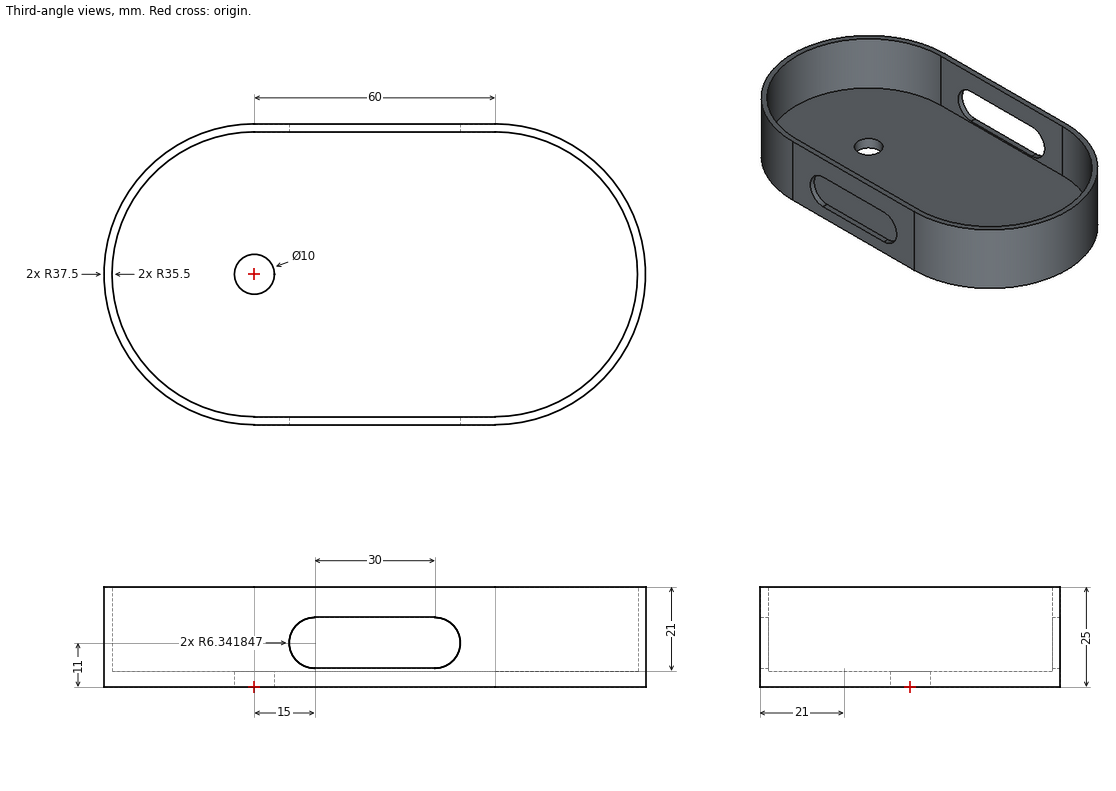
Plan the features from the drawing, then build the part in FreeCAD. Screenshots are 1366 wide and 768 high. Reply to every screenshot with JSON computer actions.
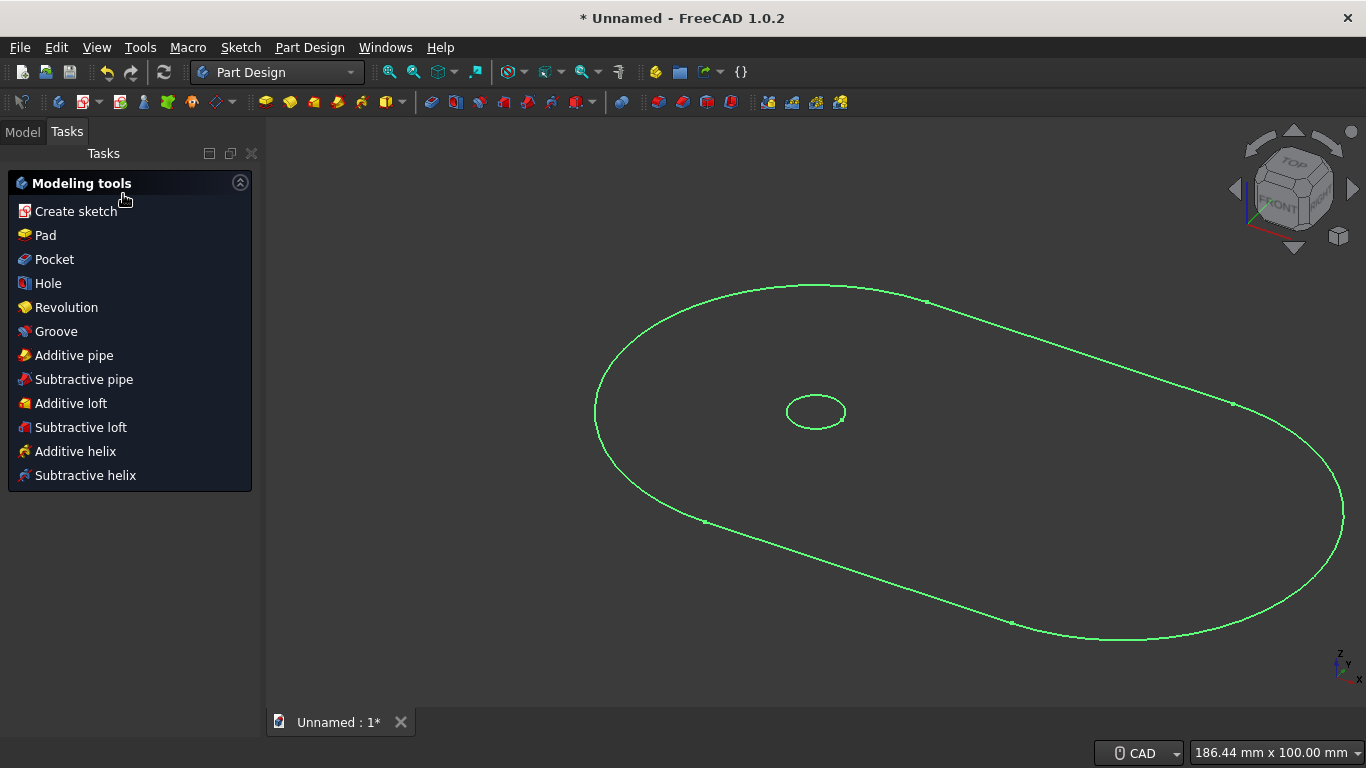
{"action": "left_click", "coordinate": [266, 102]}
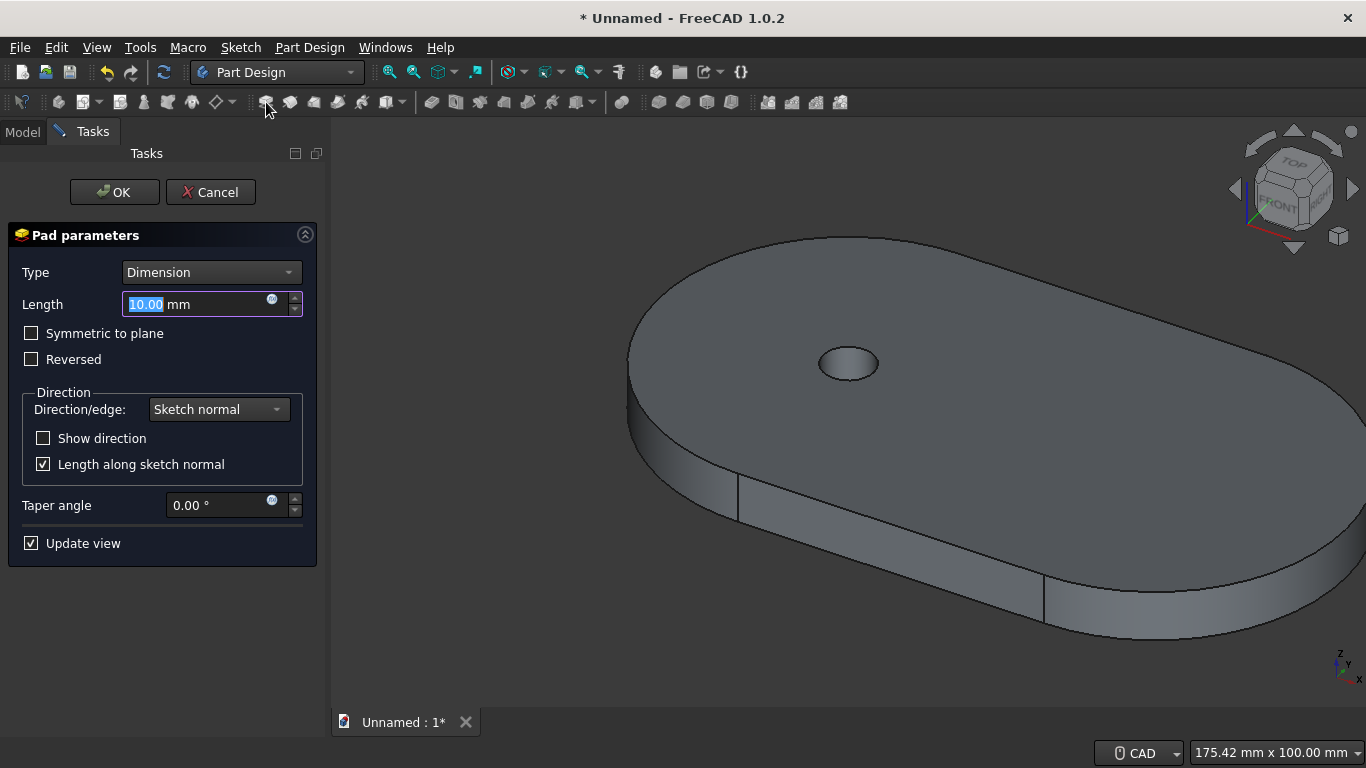
{"action": "type", "text": "25"}
{"action": "key", "text": "Tab"}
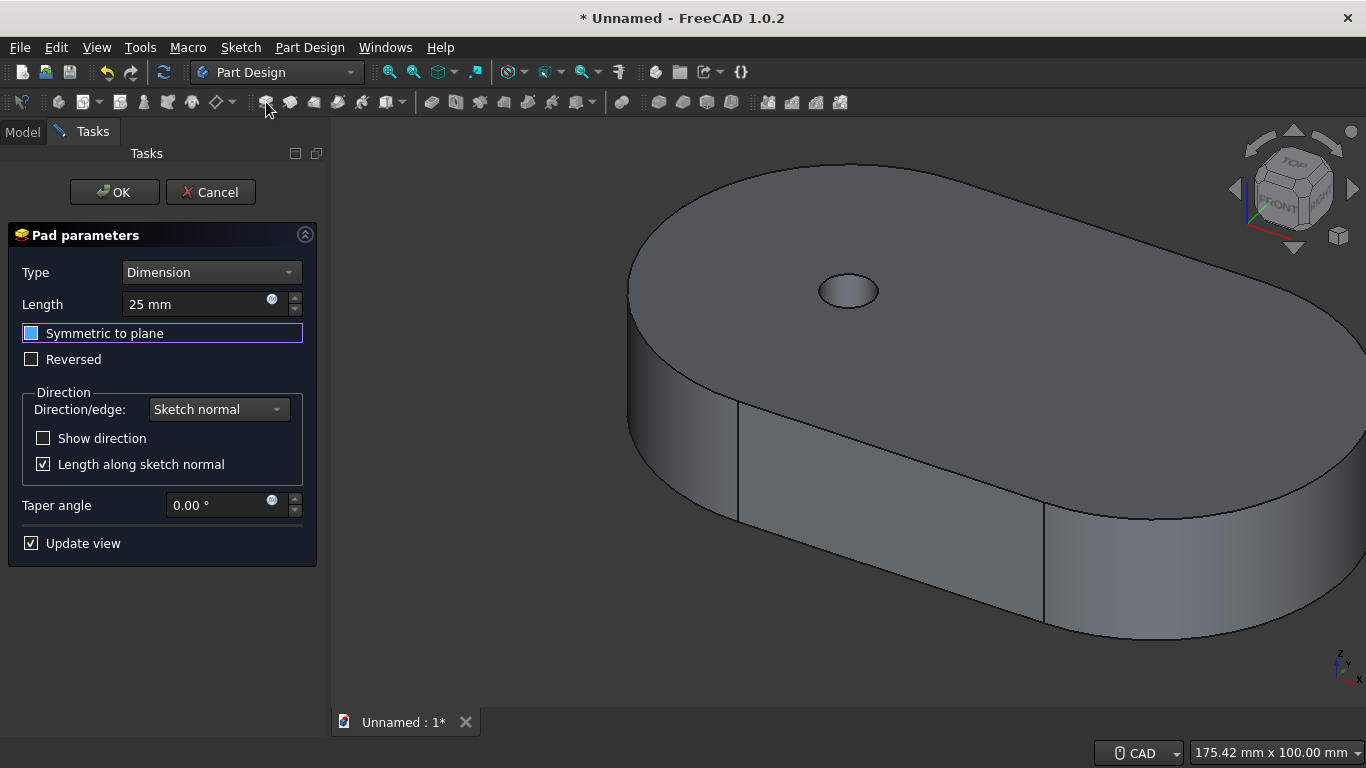
{"action": "left_click", "coordinate": [115, 192]}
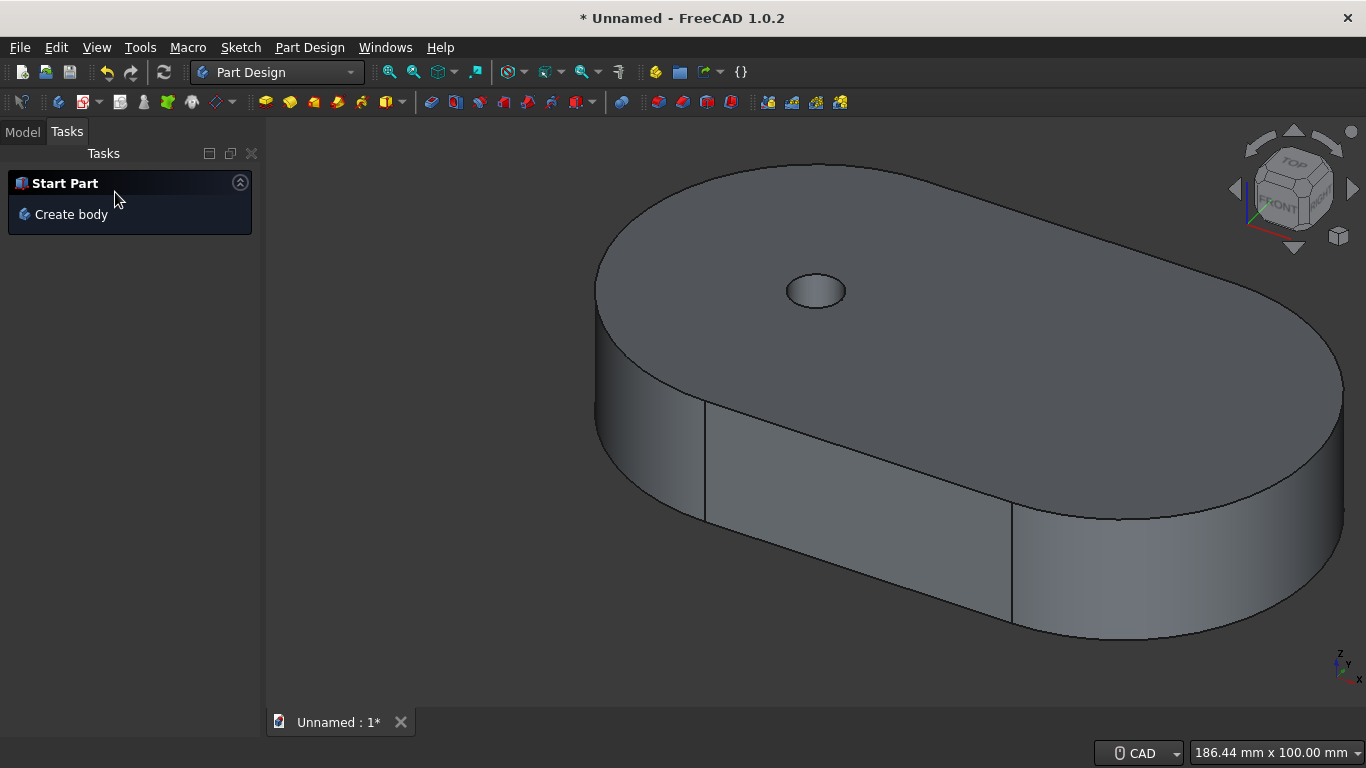
{"action": "left_click", "coordinate": [390, 72]}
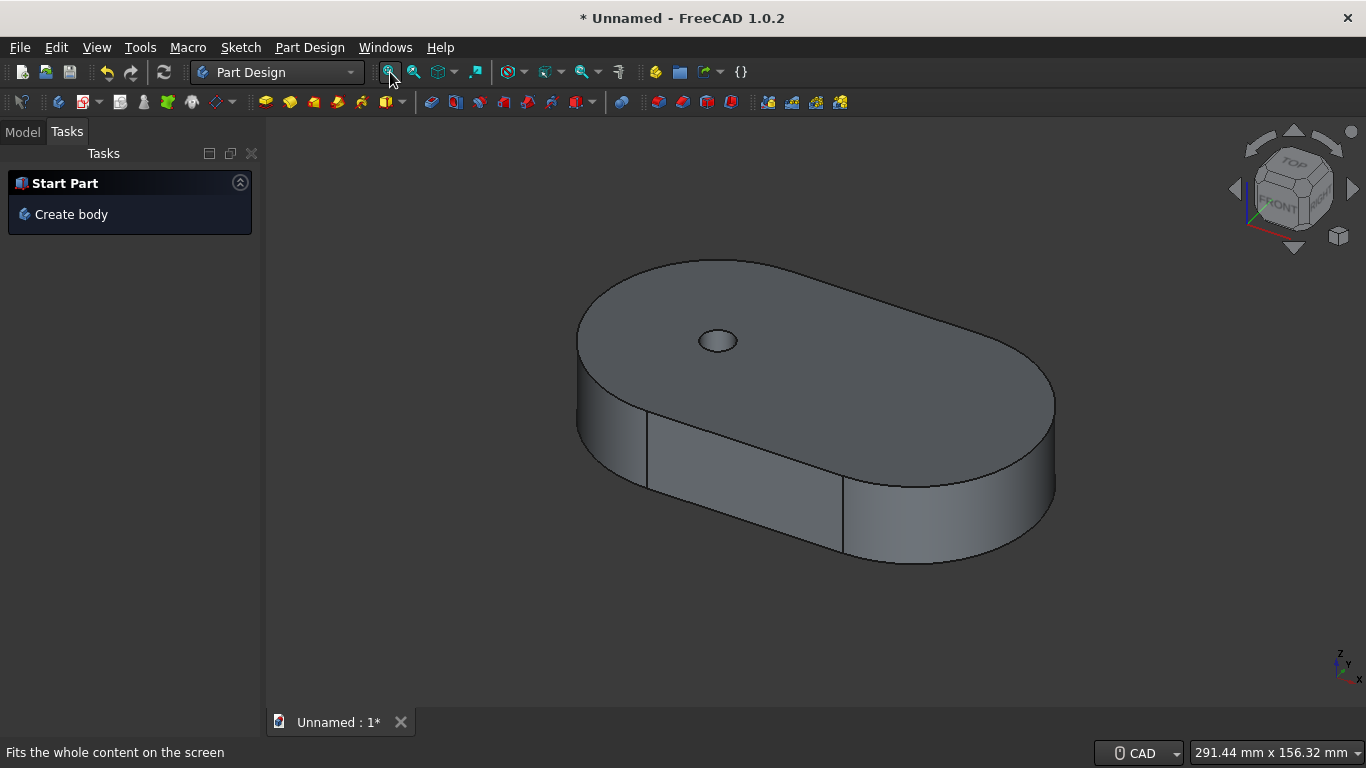
{"action": "left_click", "coordinate": [879, 393]}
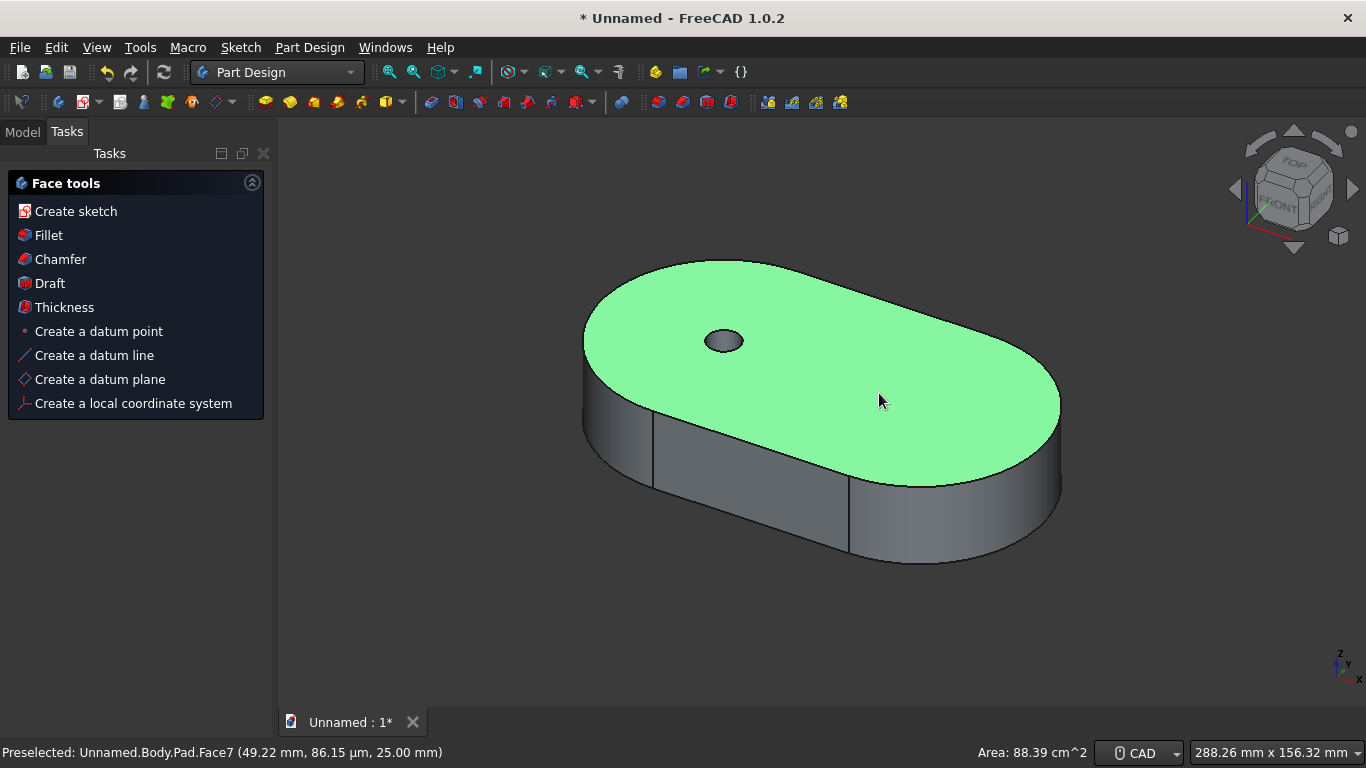
{"action": "left_click", "coordinate": [84, 102]}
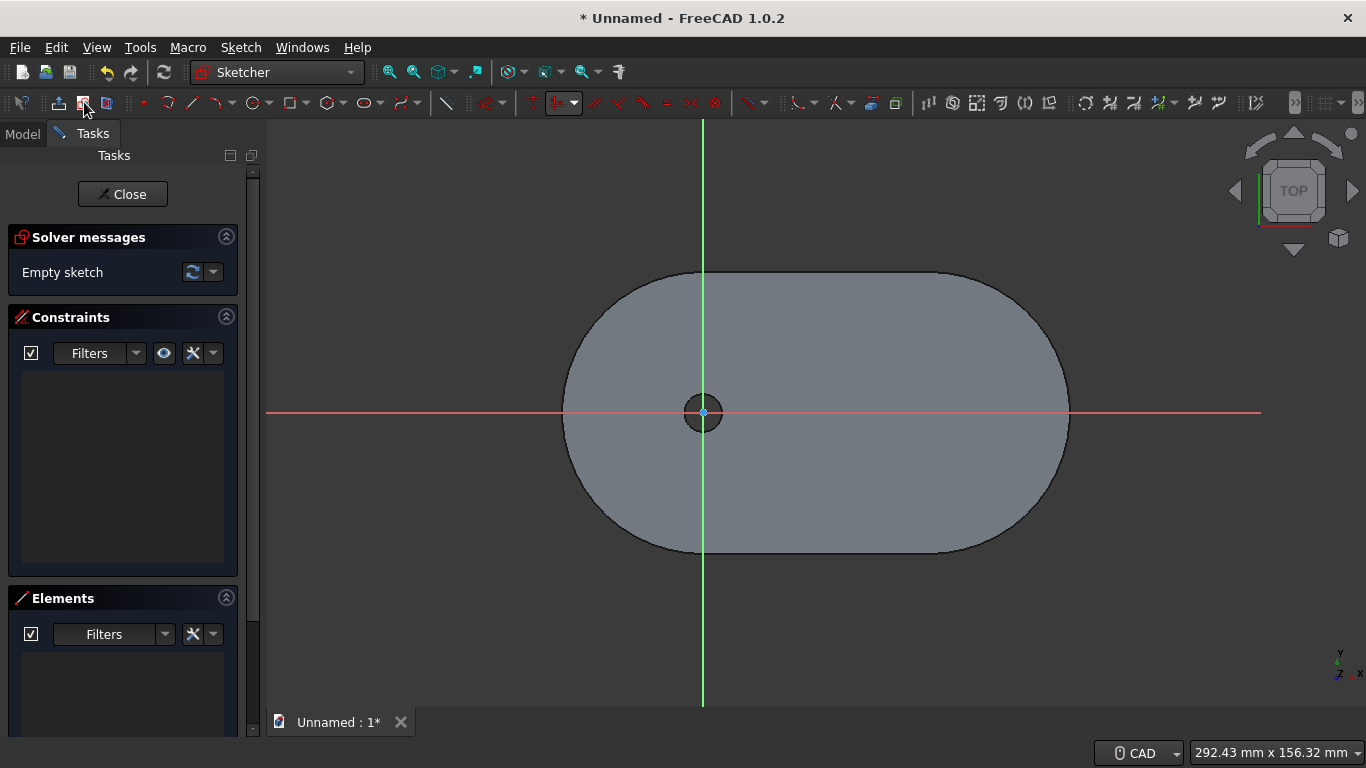
{"action": "left_click", "coordinate": [364, 104]}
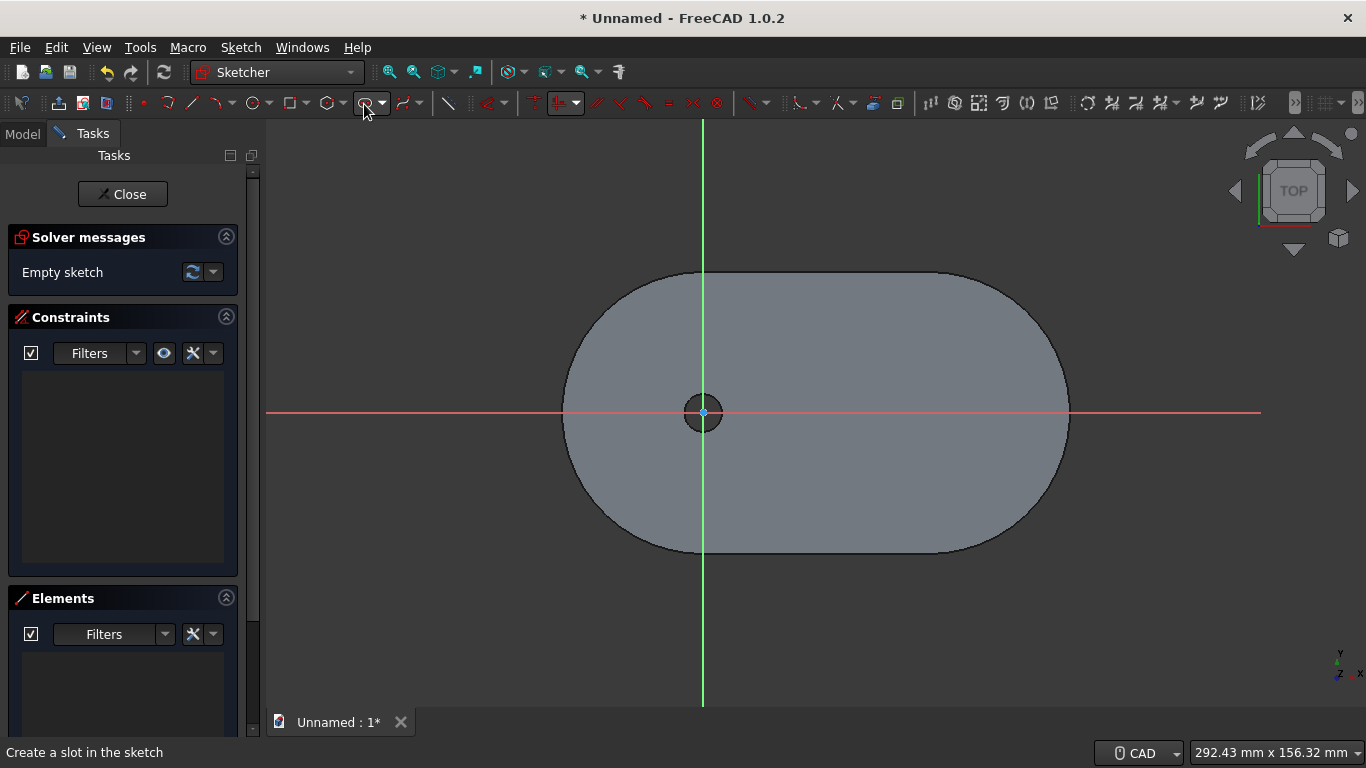
{"action": "left_click", "coordinate": [703, 413]}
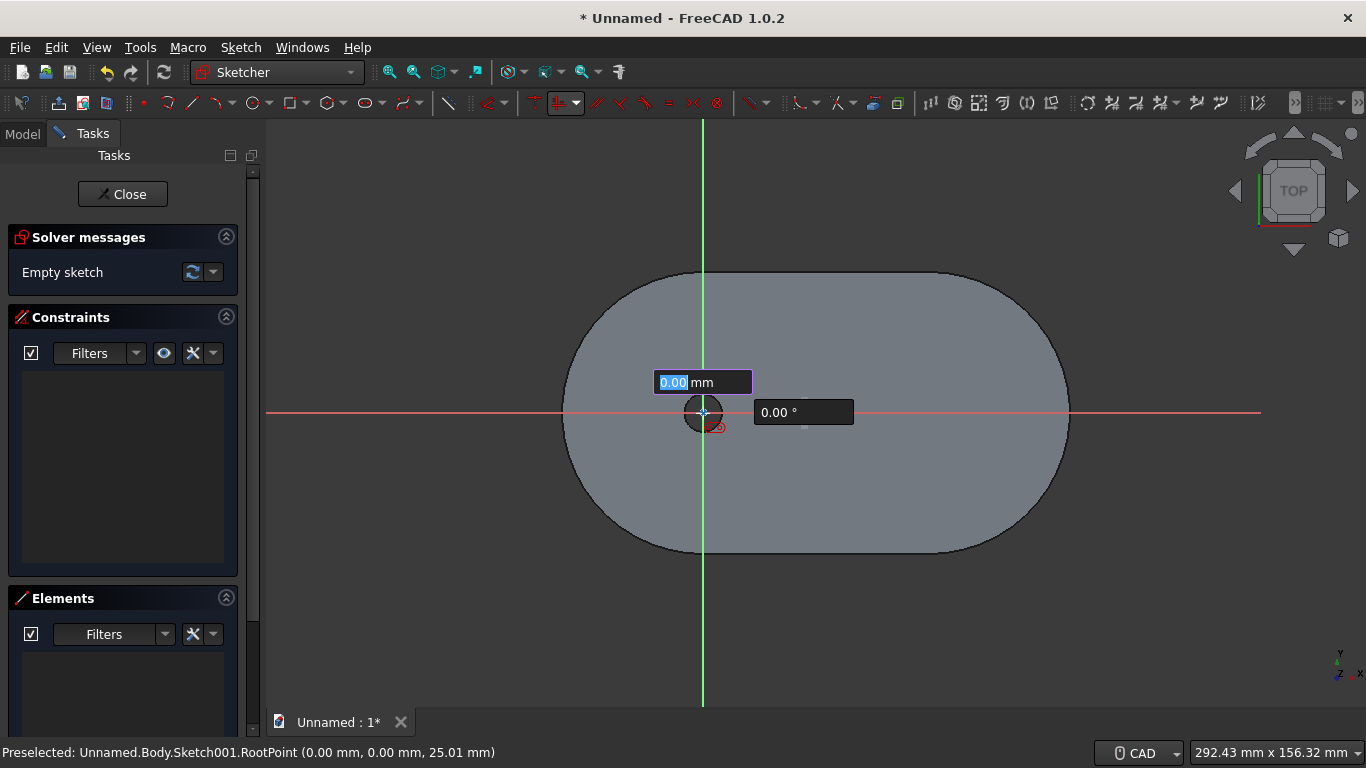
{"action": "left_click", "coordinate": [929, 404]}